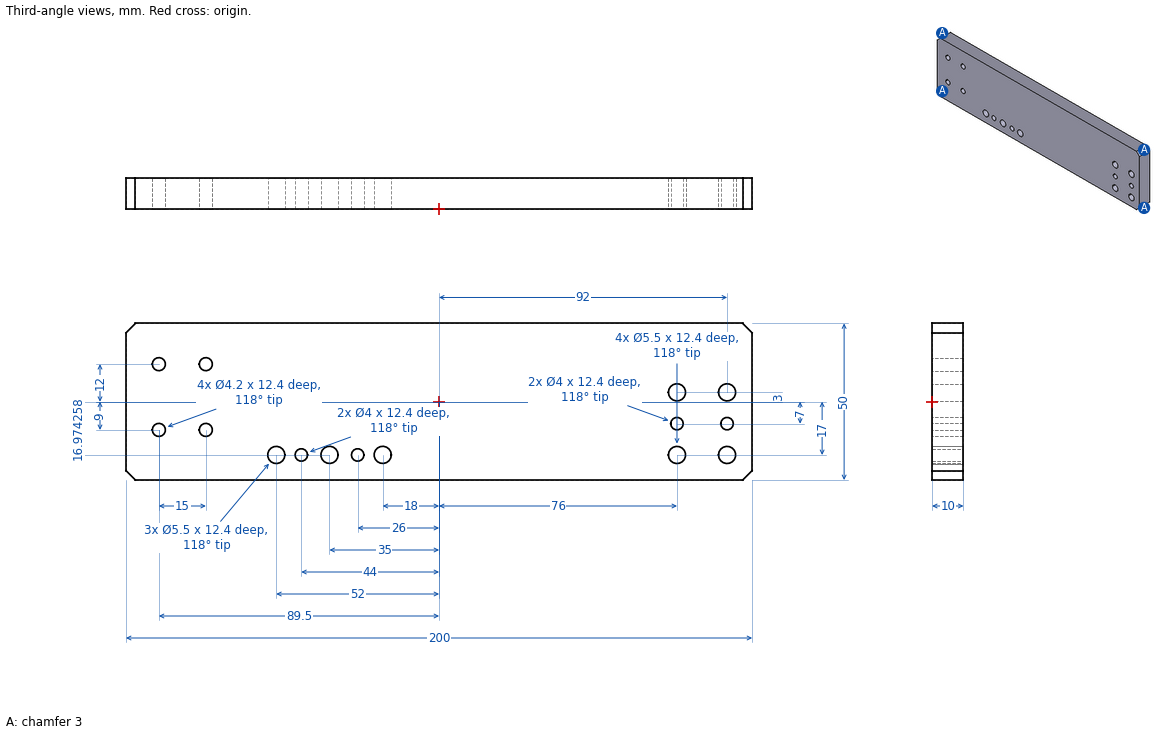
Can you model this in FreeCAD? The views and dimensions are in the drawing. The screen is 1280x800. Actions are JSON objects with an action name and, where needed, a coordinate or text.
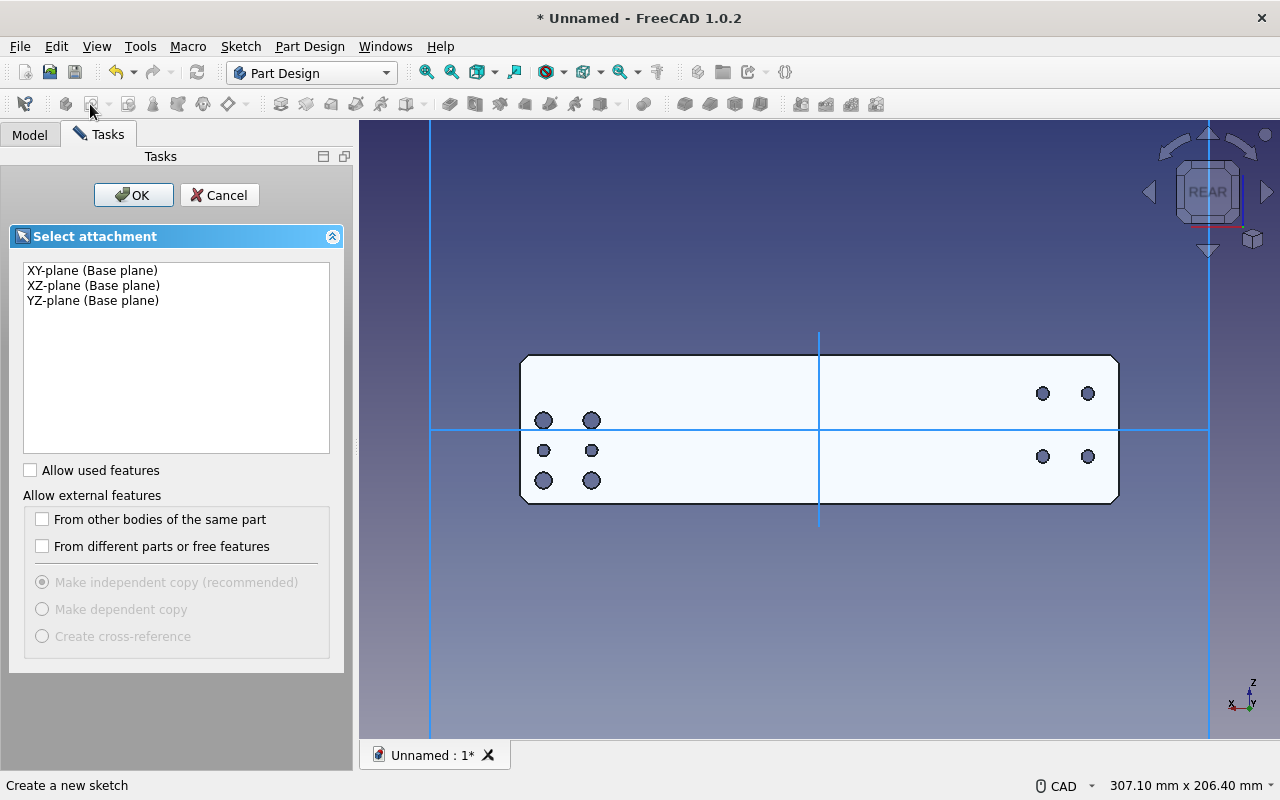
{"action": "left_click", "coordinate": [84, 286]}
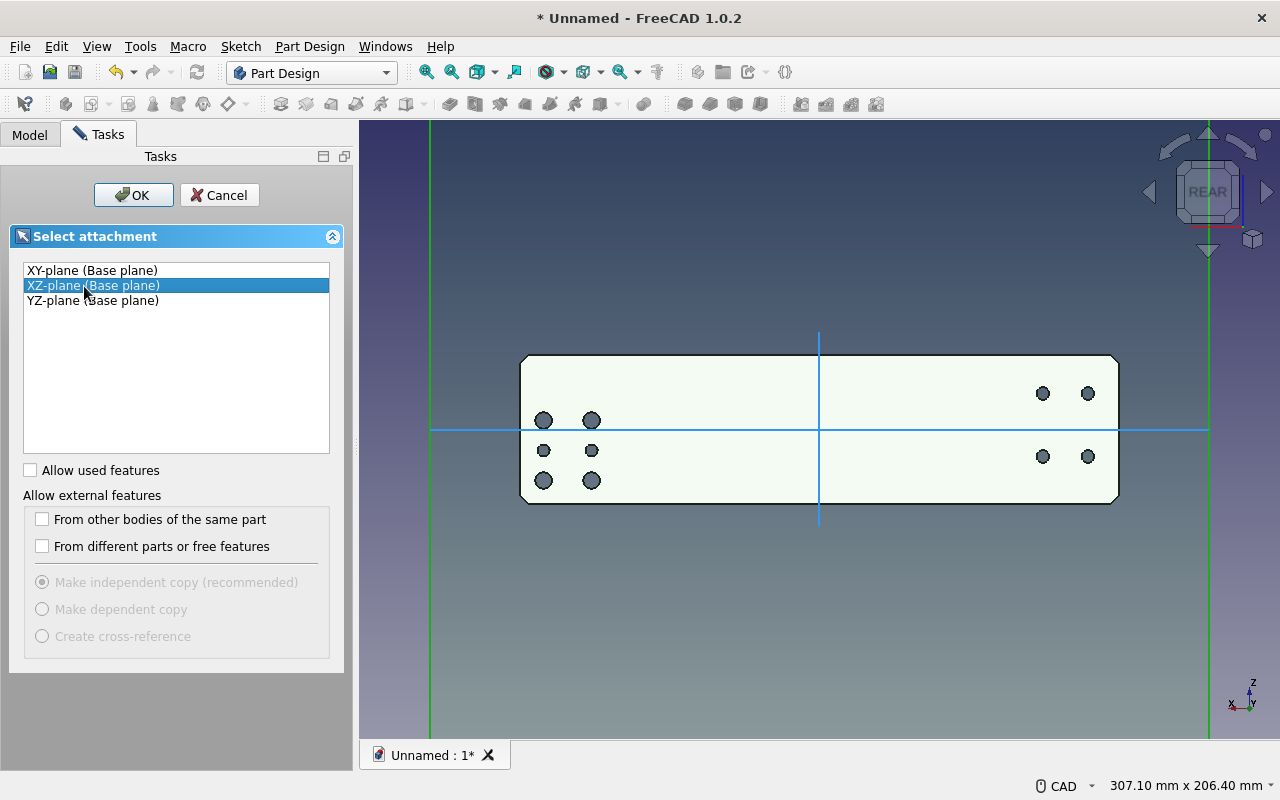
{"action": "left_click", "coordinate": [134, 195]}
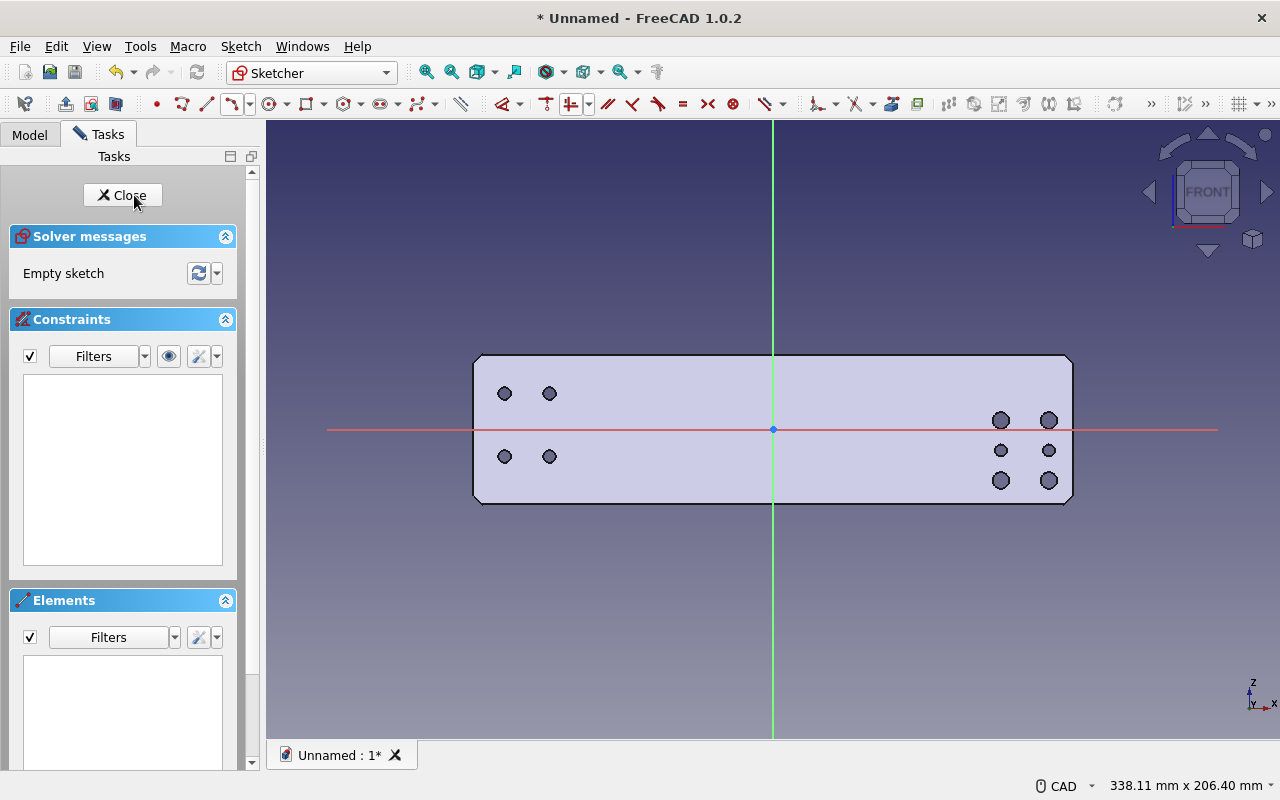
{"action": "scroll", "coordinate": [685, 472], "scroll_direction": "up", "scroll_amount": 6}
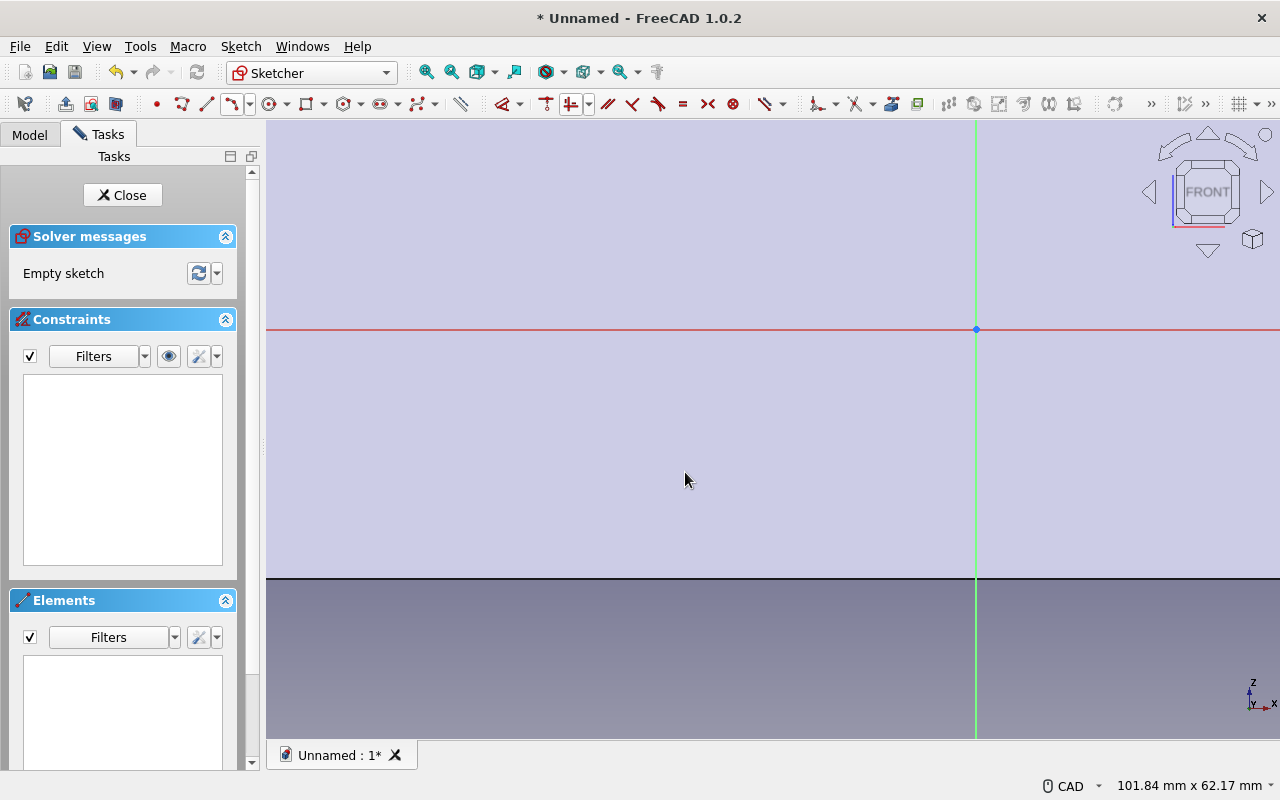
{"action": "key", "text": "g c"}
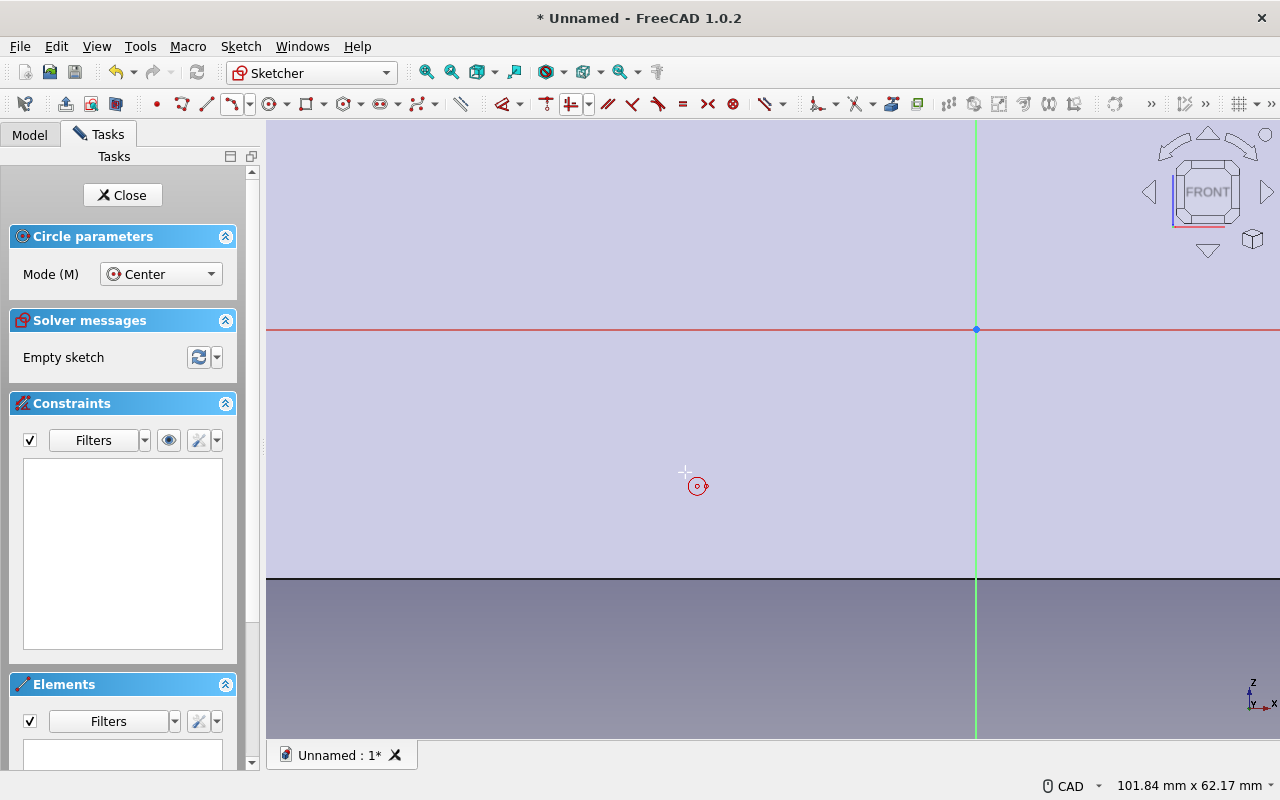
{"action": "left_click", "coordinate": [458, 499]}
{"action": "left_click", "coordinate": [478, 479]}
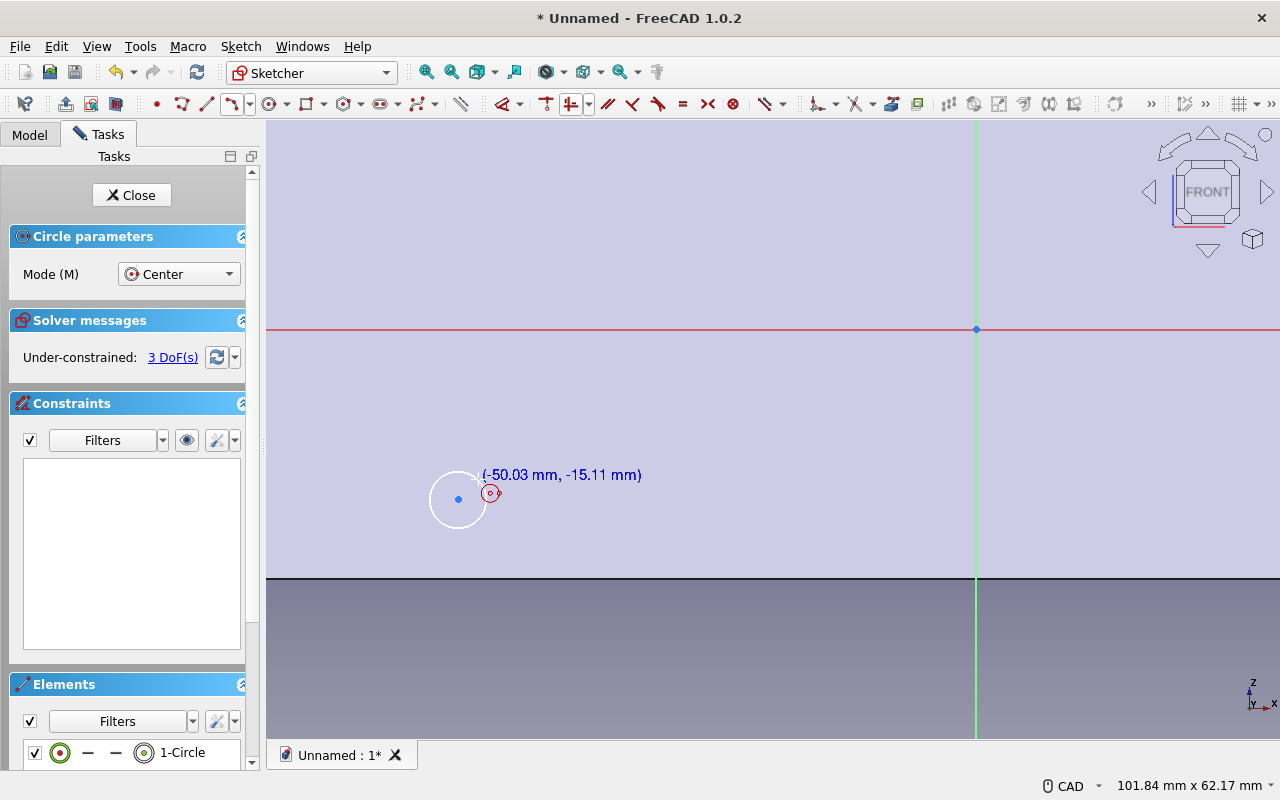
{"action": "left_click", "coordinate": [628, 499]}
{"action": "left_click", "coordinate": [647, 479]}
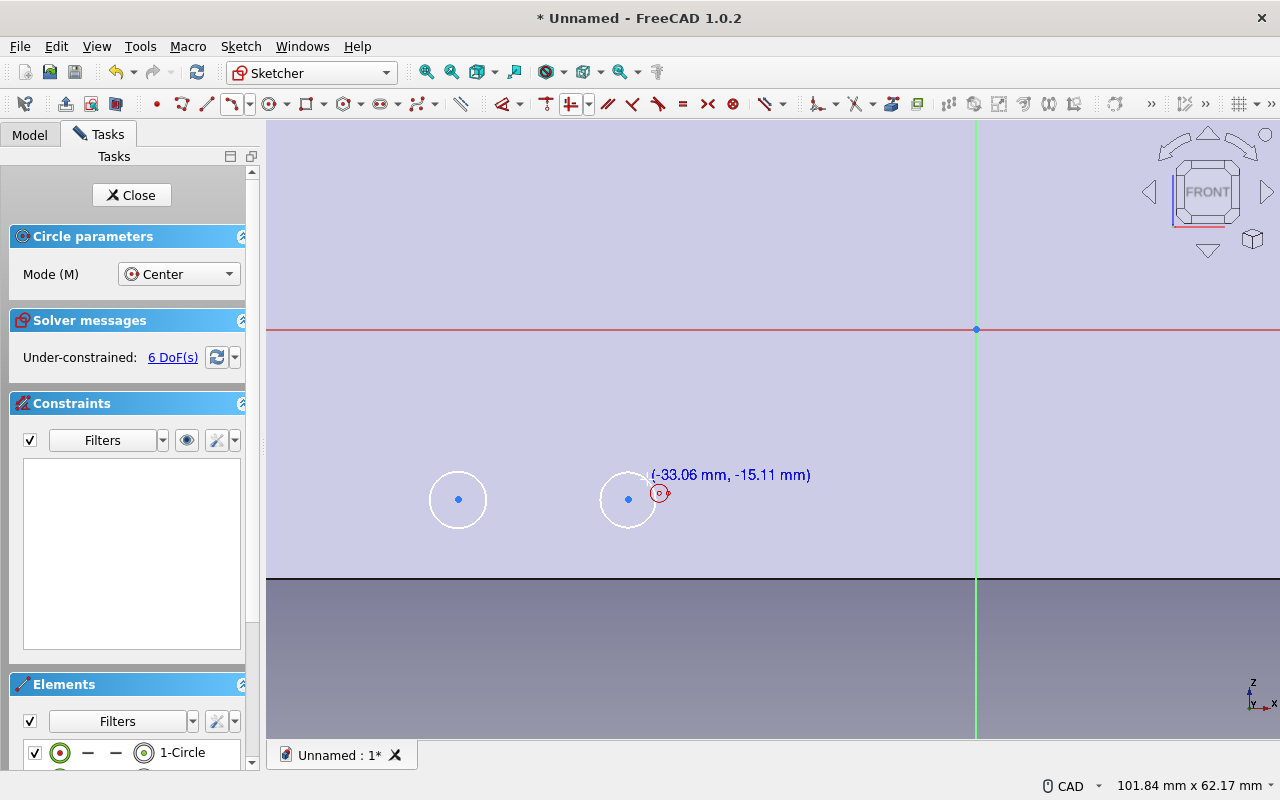
{"action": "left_click", "coordinate": [797, 499]}
{"action": "left_click", "coordinate": [816, 479]}
{"action": "key", "text": "Escape"}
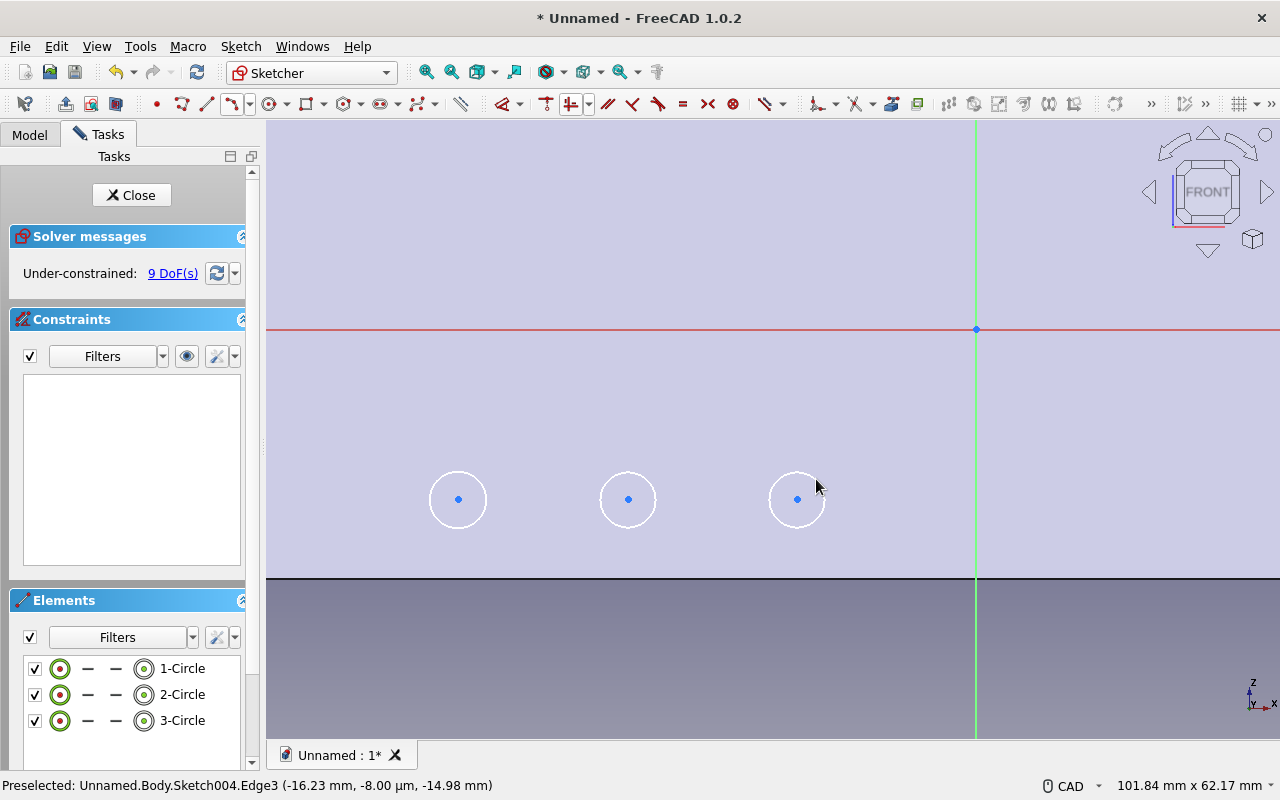
{"action": "left_click", "coordinate": [478, 480]}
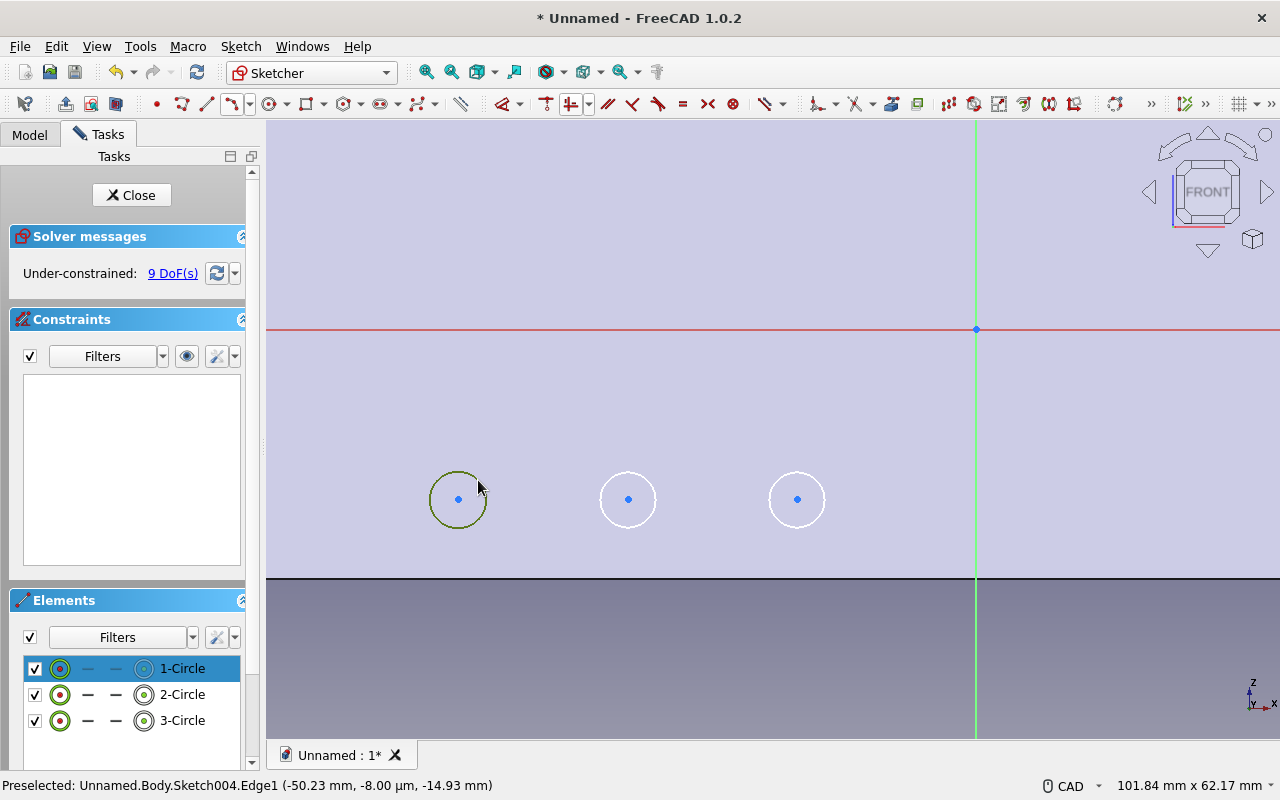
{"action": "left_click", "coordinate": [647, 480]}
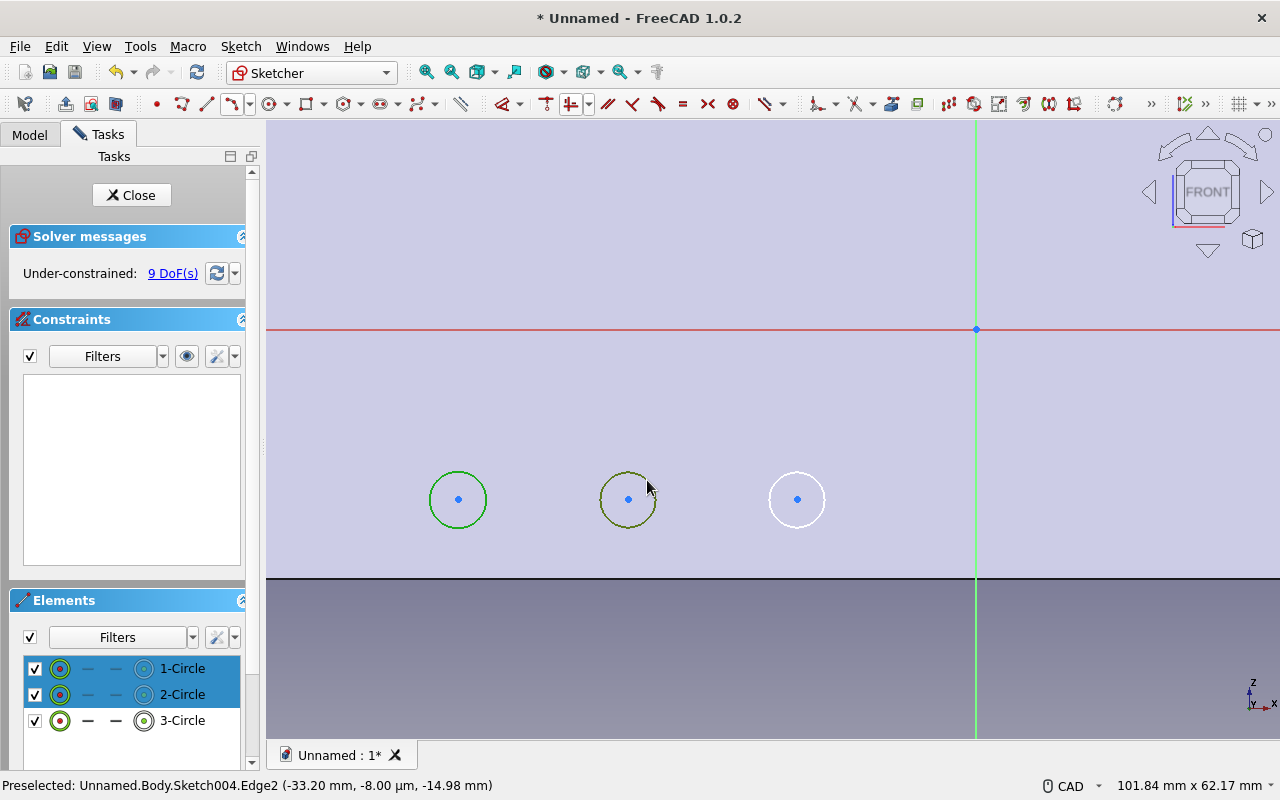
{"action": "left_click", "coordinate": [816, 480]}